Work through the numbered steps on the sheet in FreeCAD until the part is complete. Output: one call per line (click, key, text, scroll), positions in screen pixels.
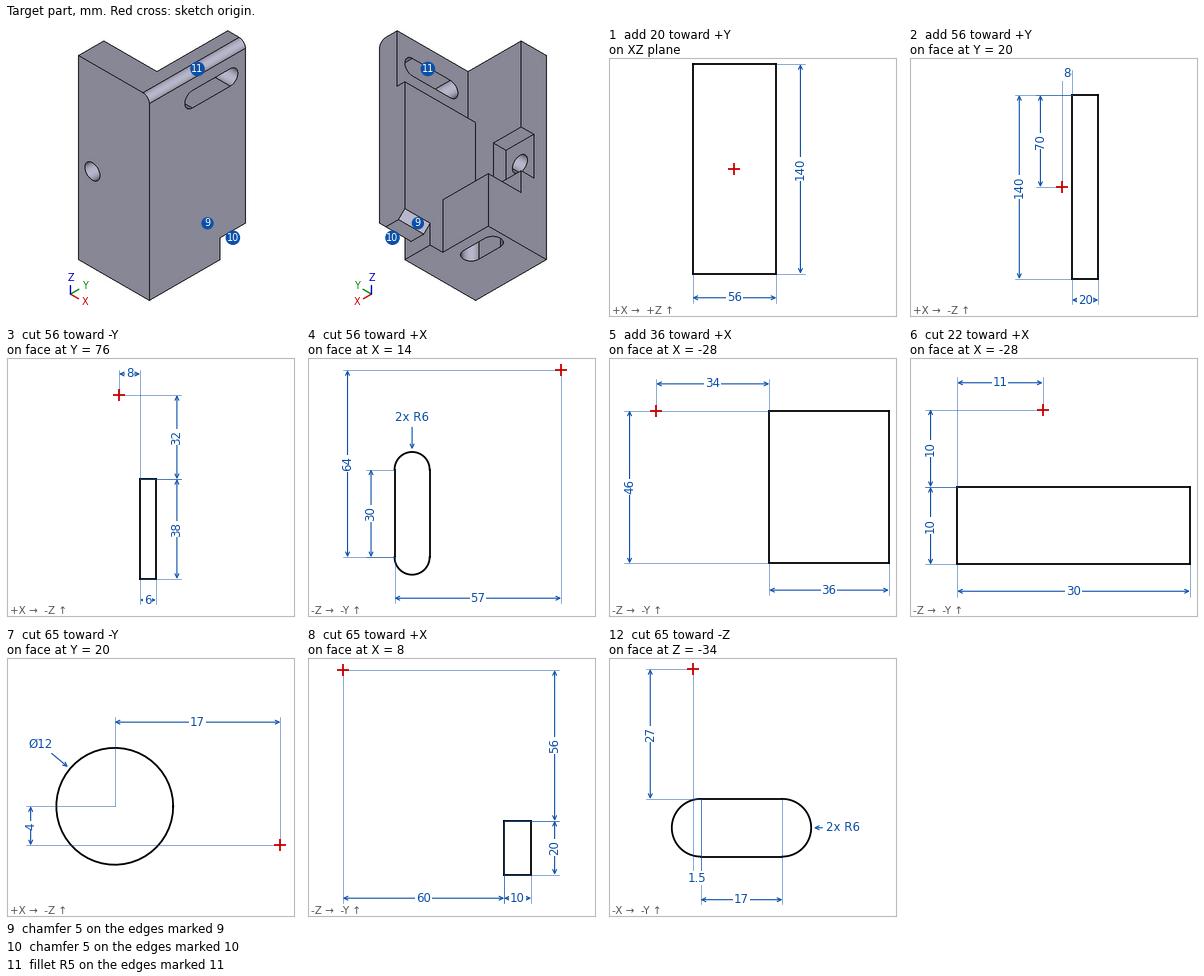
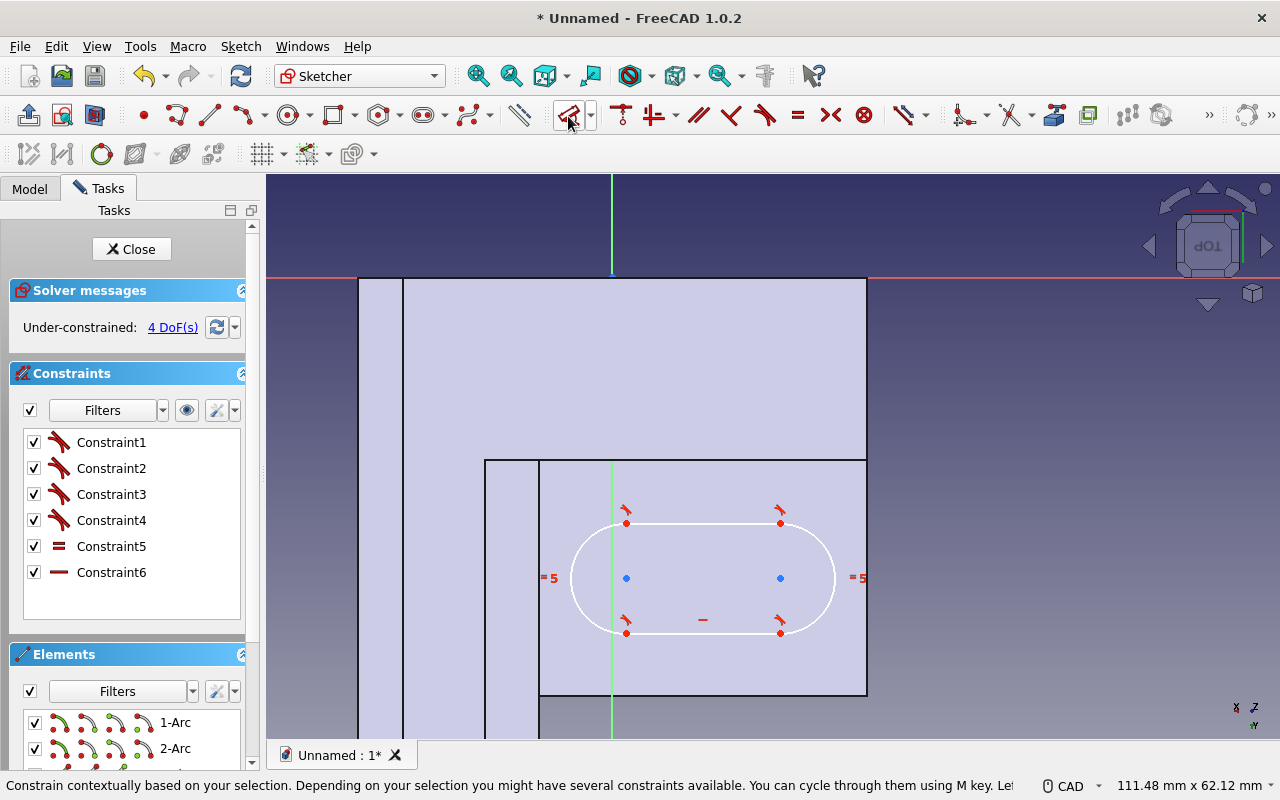
click(582, 547)
click(556, 528)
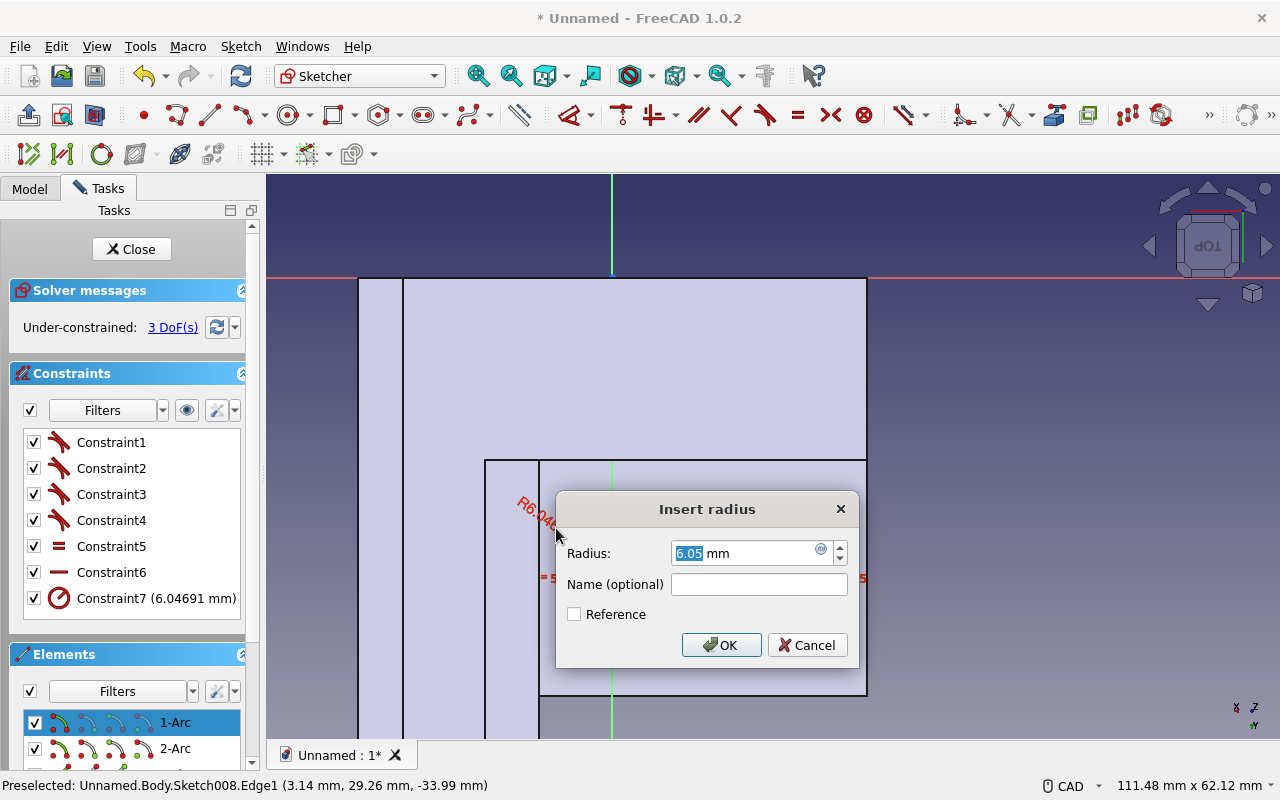
text(6)
key(Return)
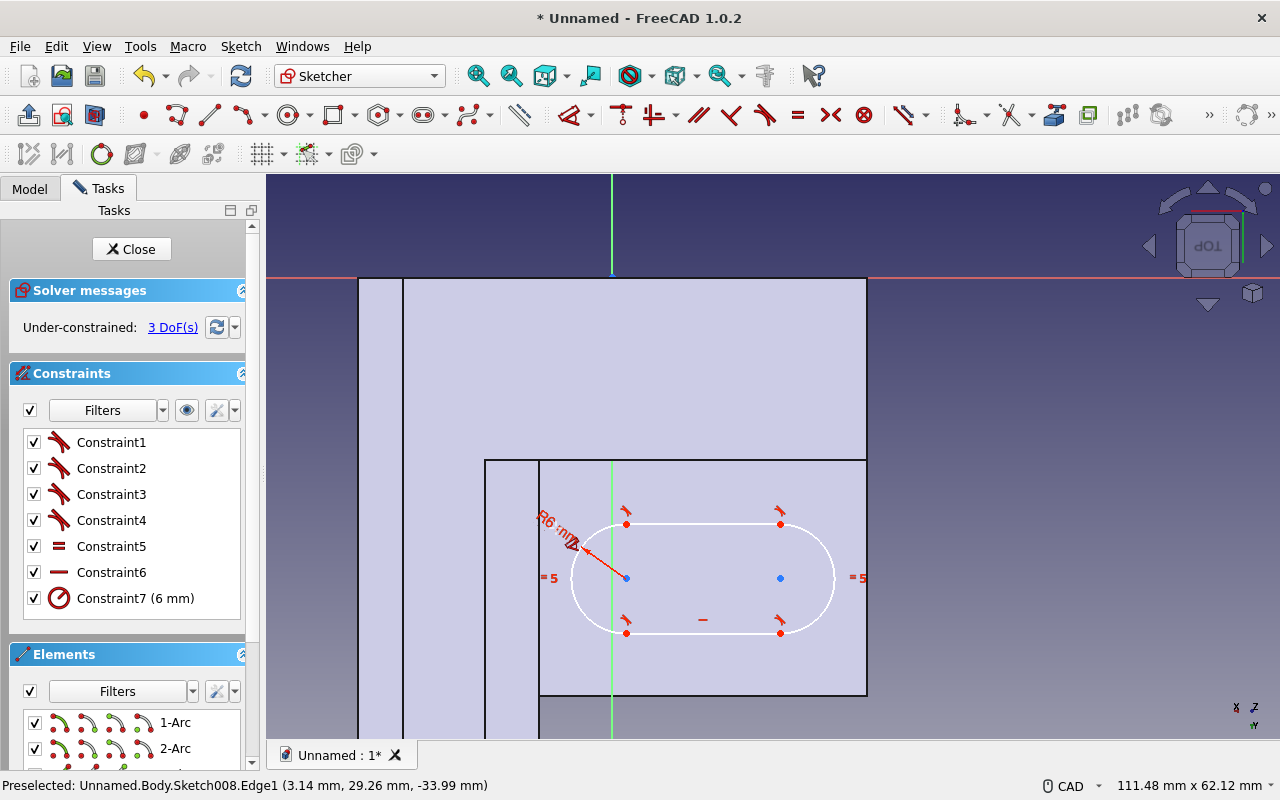
click(672, 524)
click(703, 558)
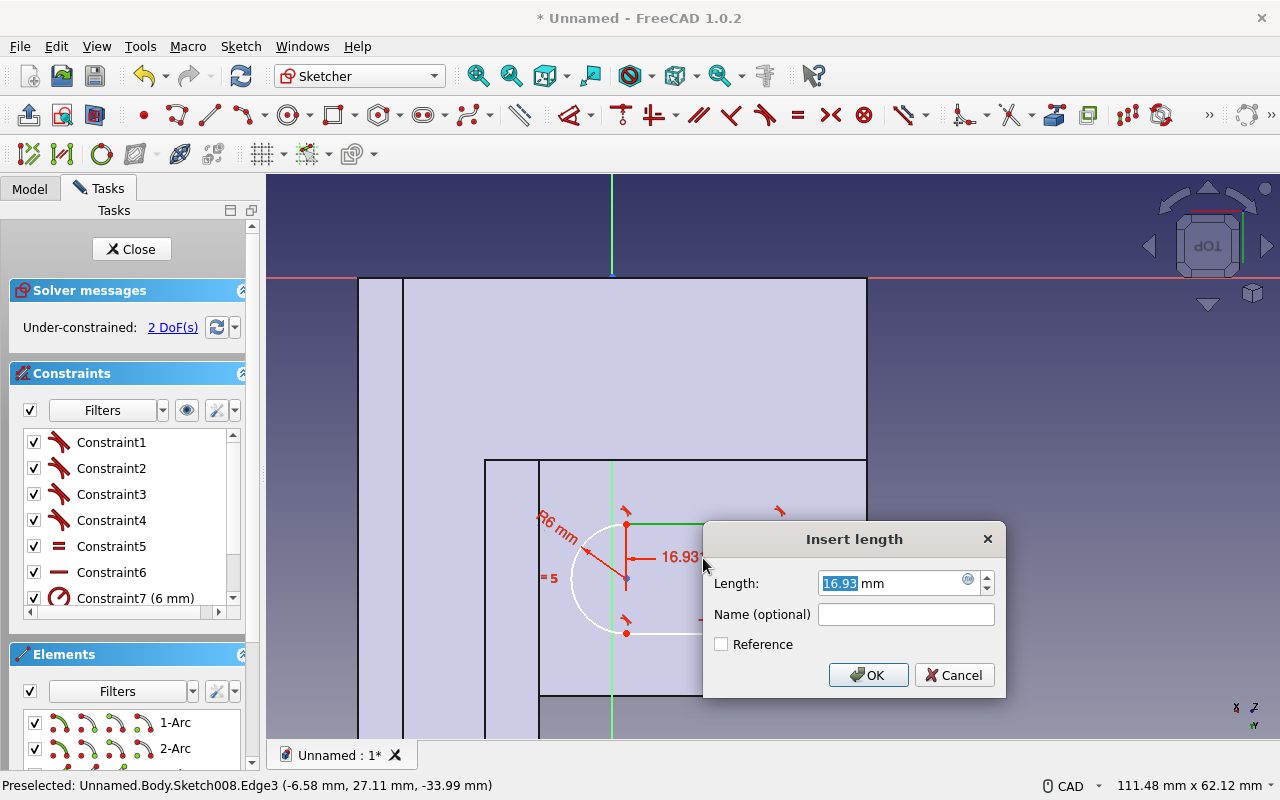
text(17)
key(Return)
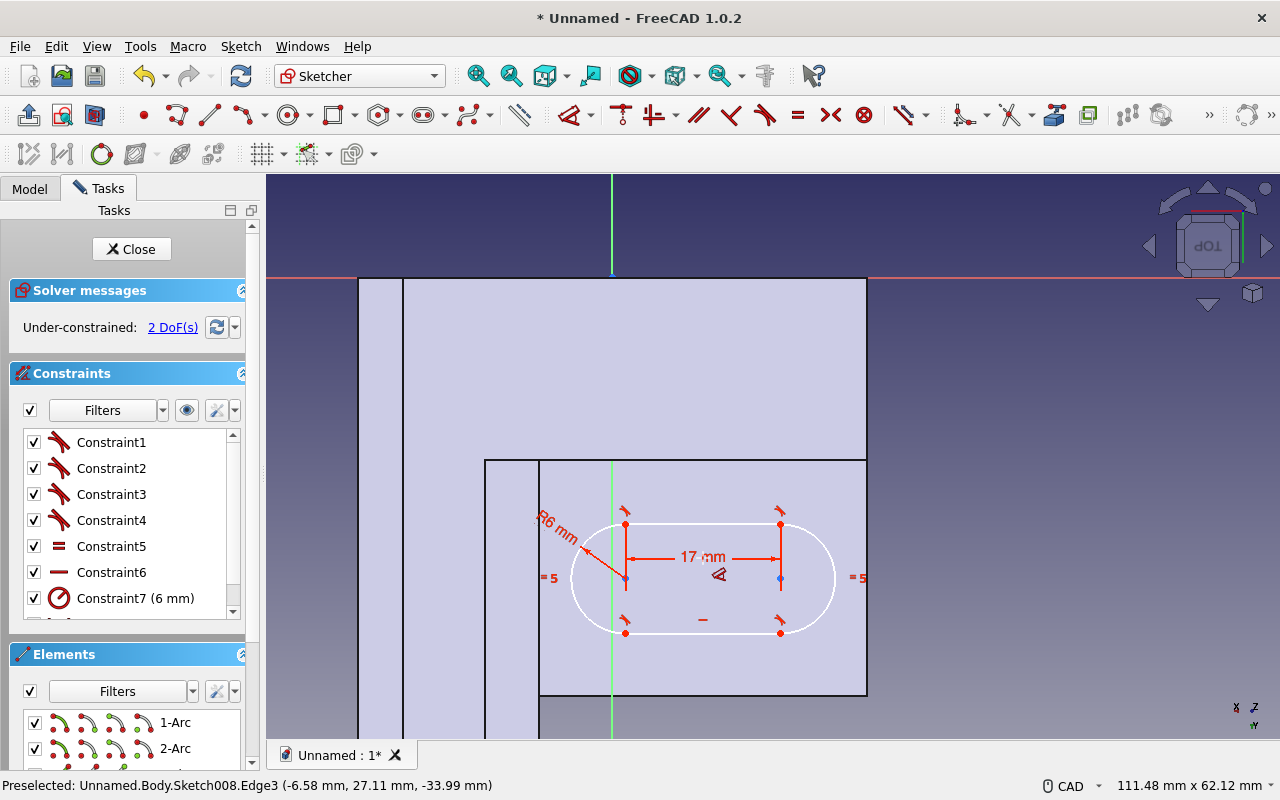
click(626, 524)
click(578, 401)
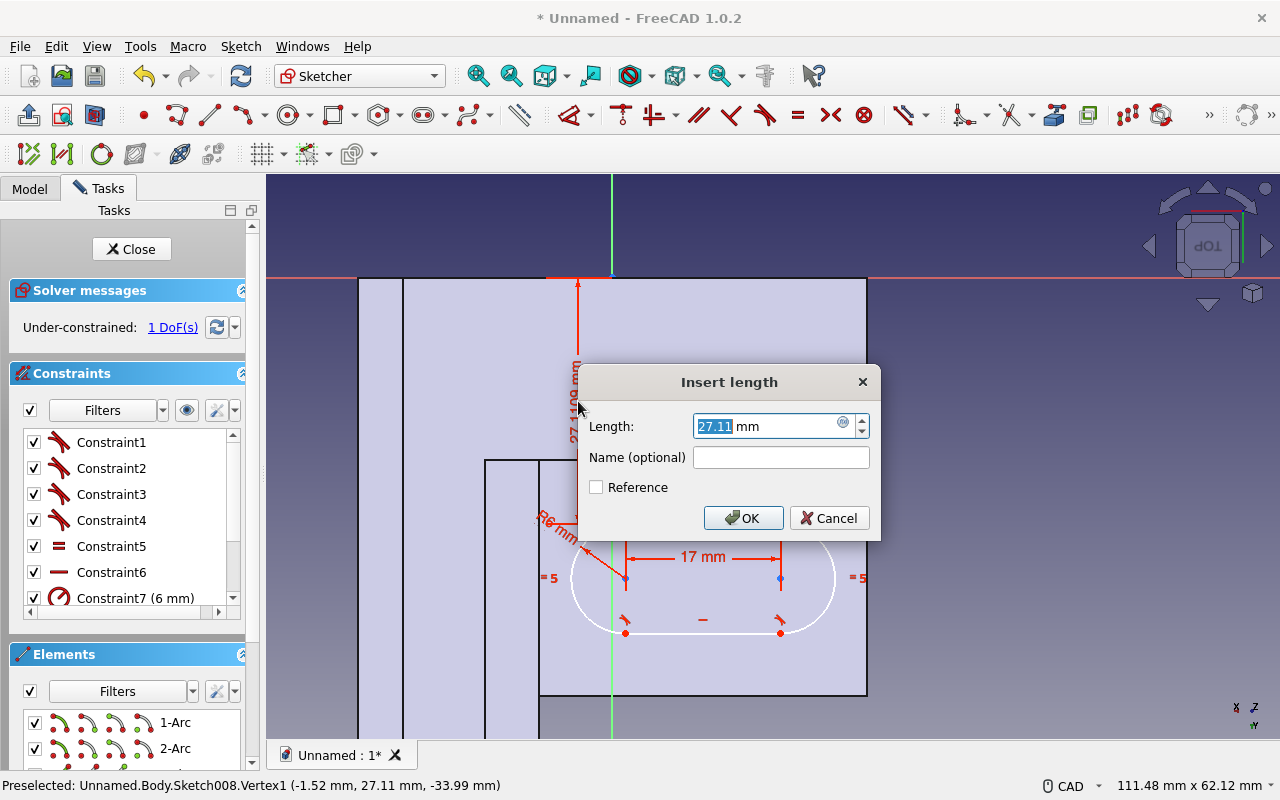
text(27)
key(Return)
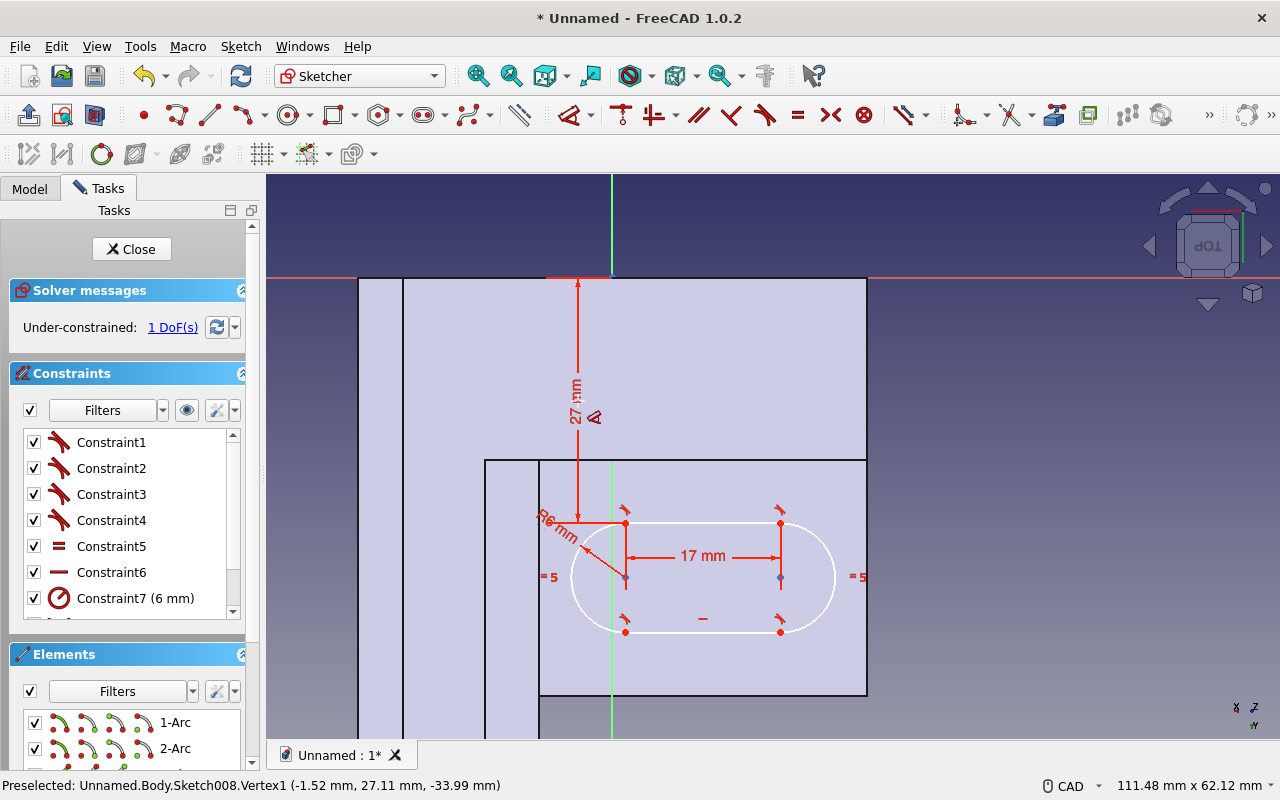
scroll(626, 523, up, 6)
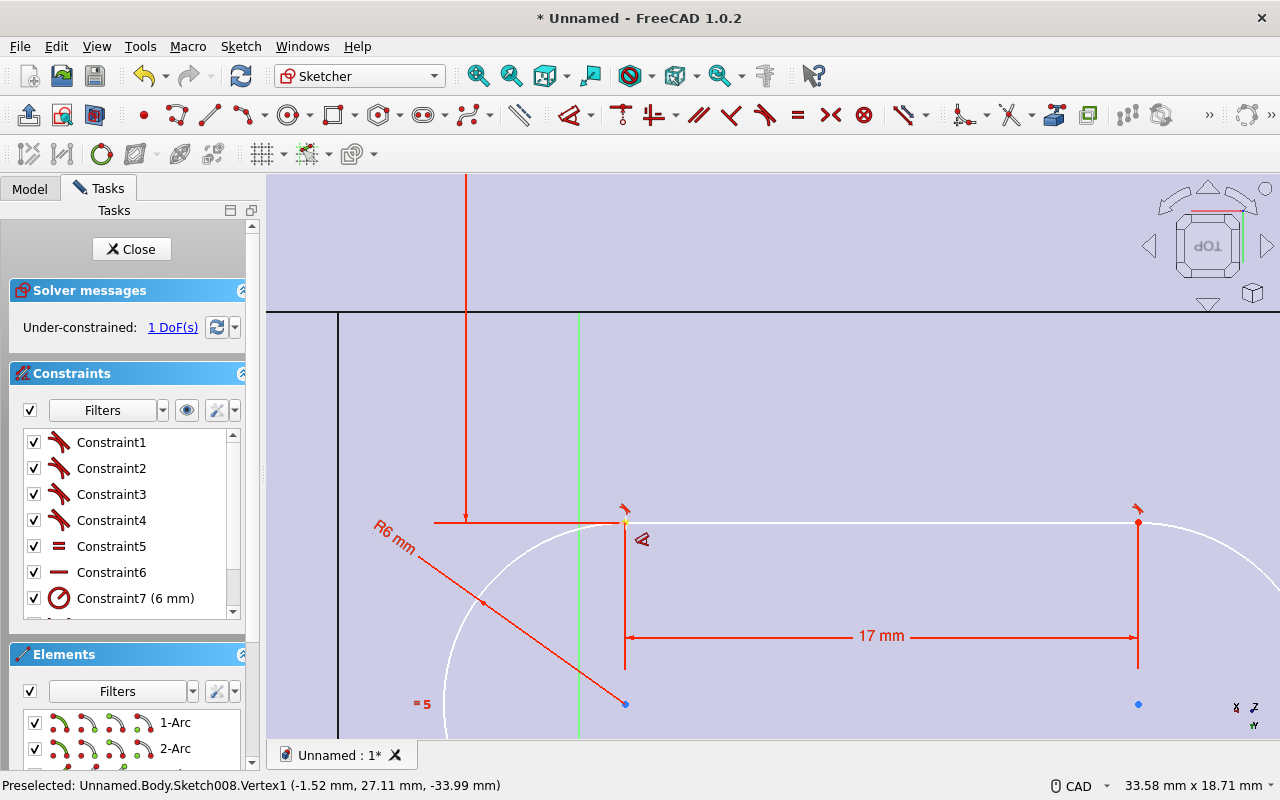
click(625, 523)
click(602, 557)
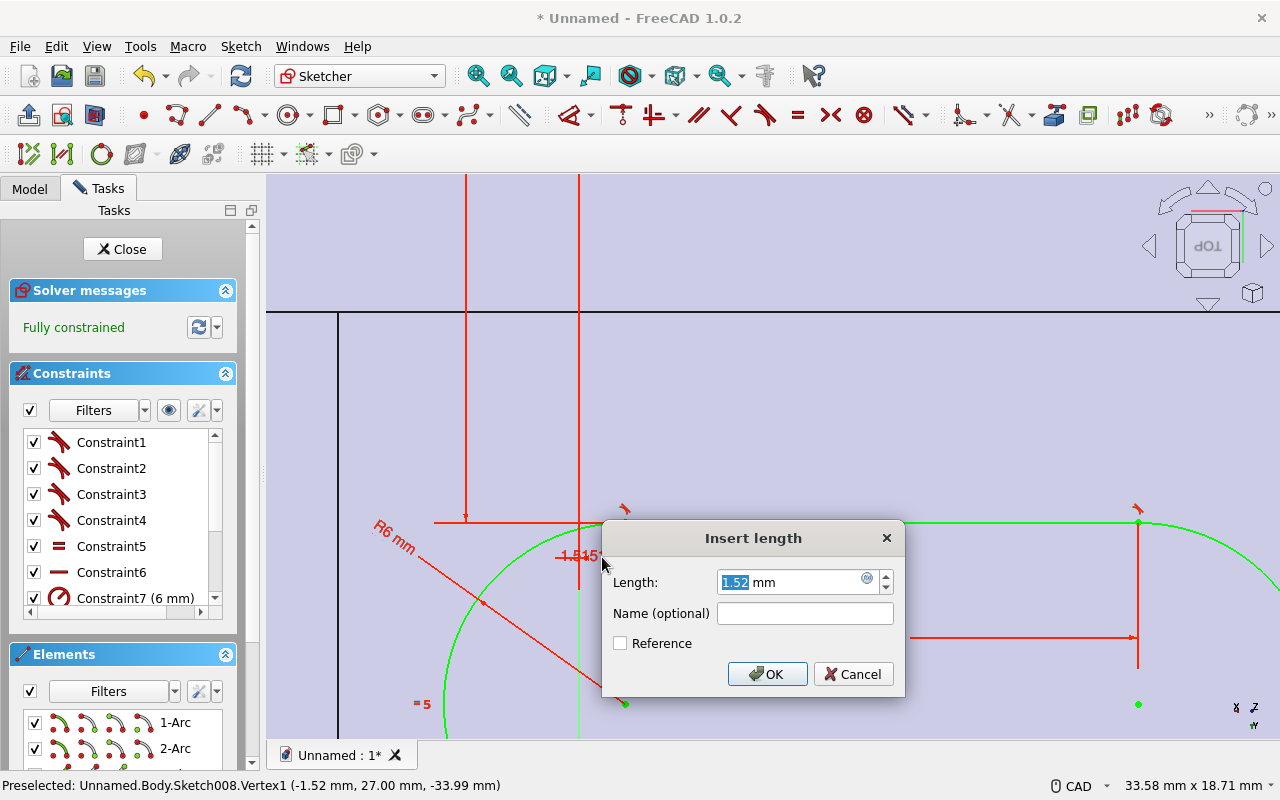
text(1.5)
key(Return)
key(Escape)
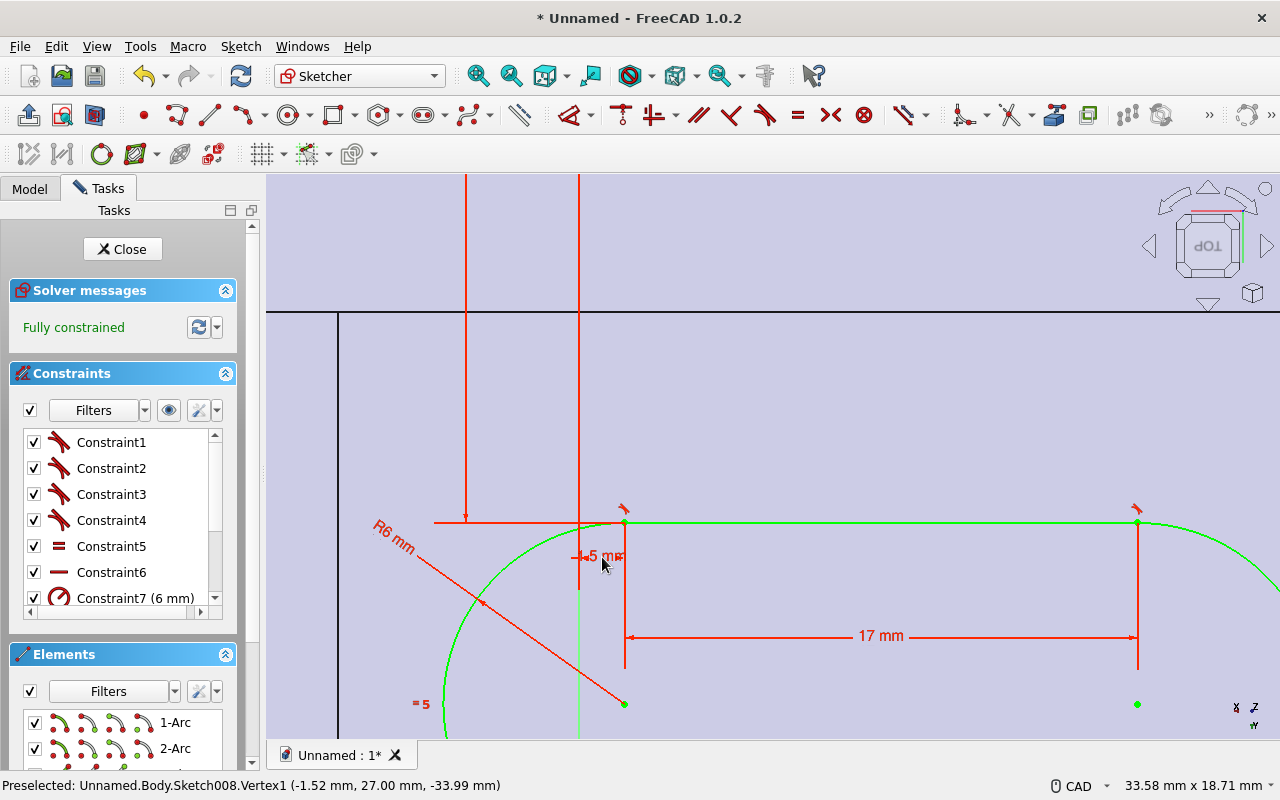
click(123, 249)